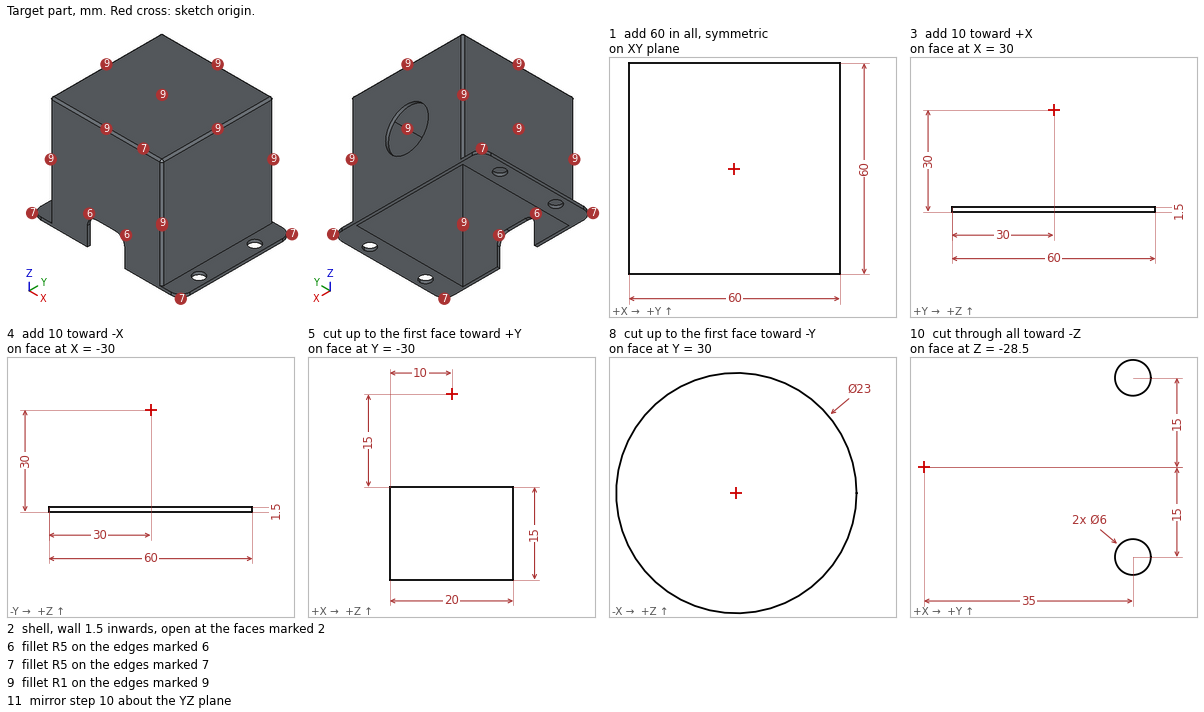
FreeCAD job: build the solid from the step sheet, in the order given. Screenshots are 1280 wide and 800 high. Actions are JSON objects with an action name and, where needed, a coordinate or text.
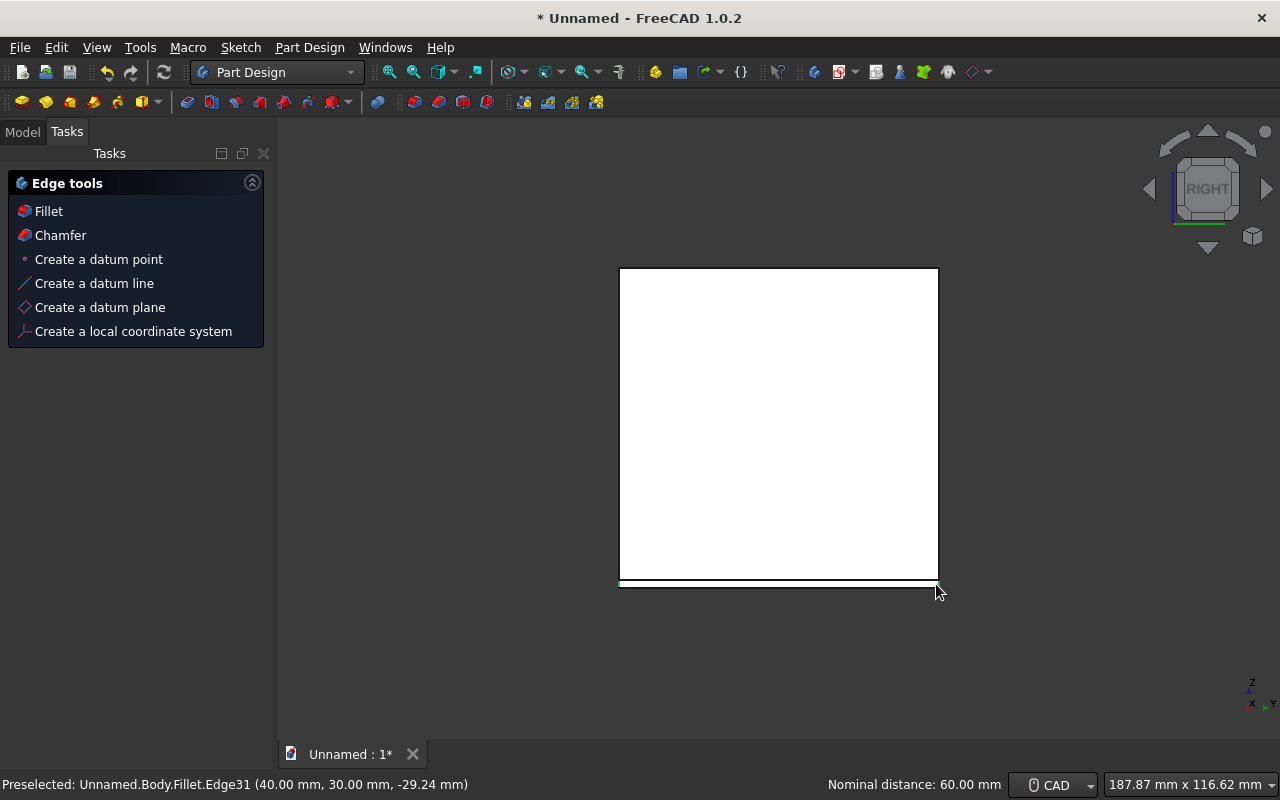
{"action": "key", "text": "5"}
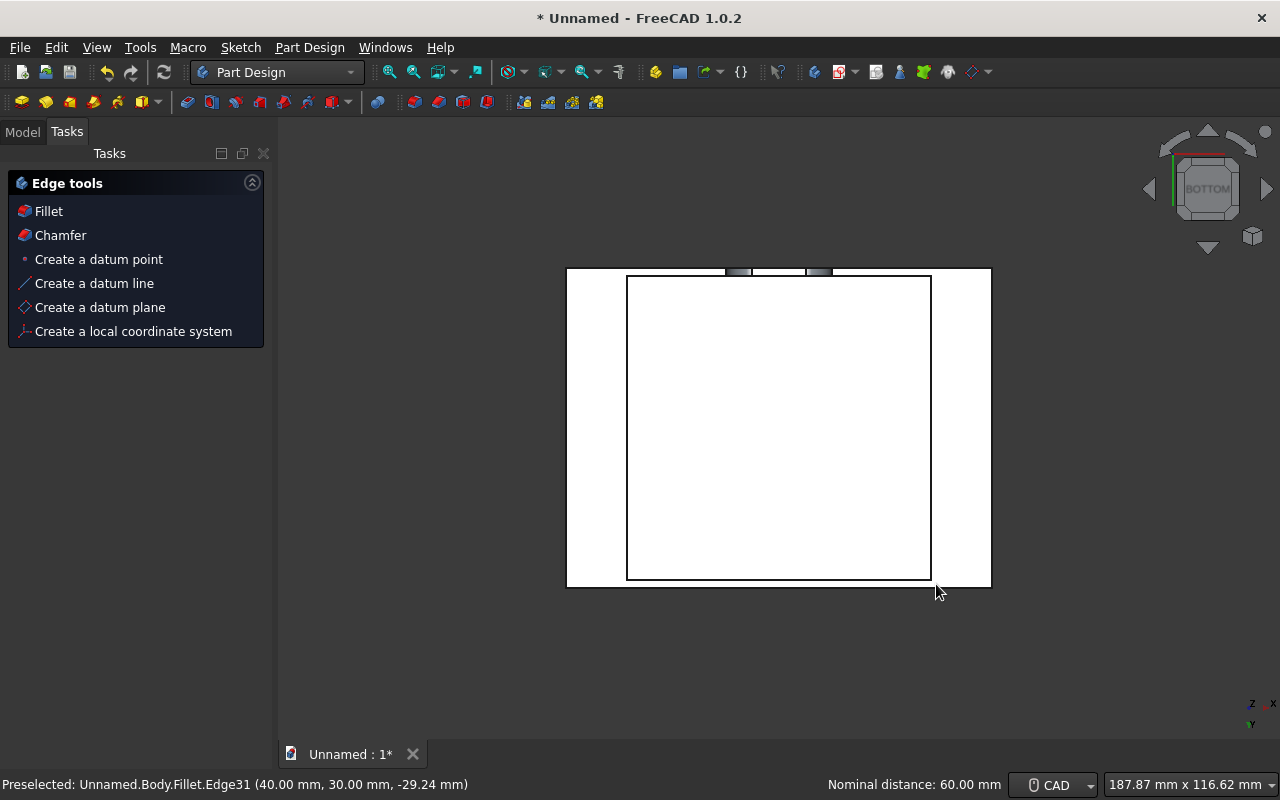
{"action": "scroll", "coordinate": [566, 267], "scroll_direction": "up", "scroll_amount": 9}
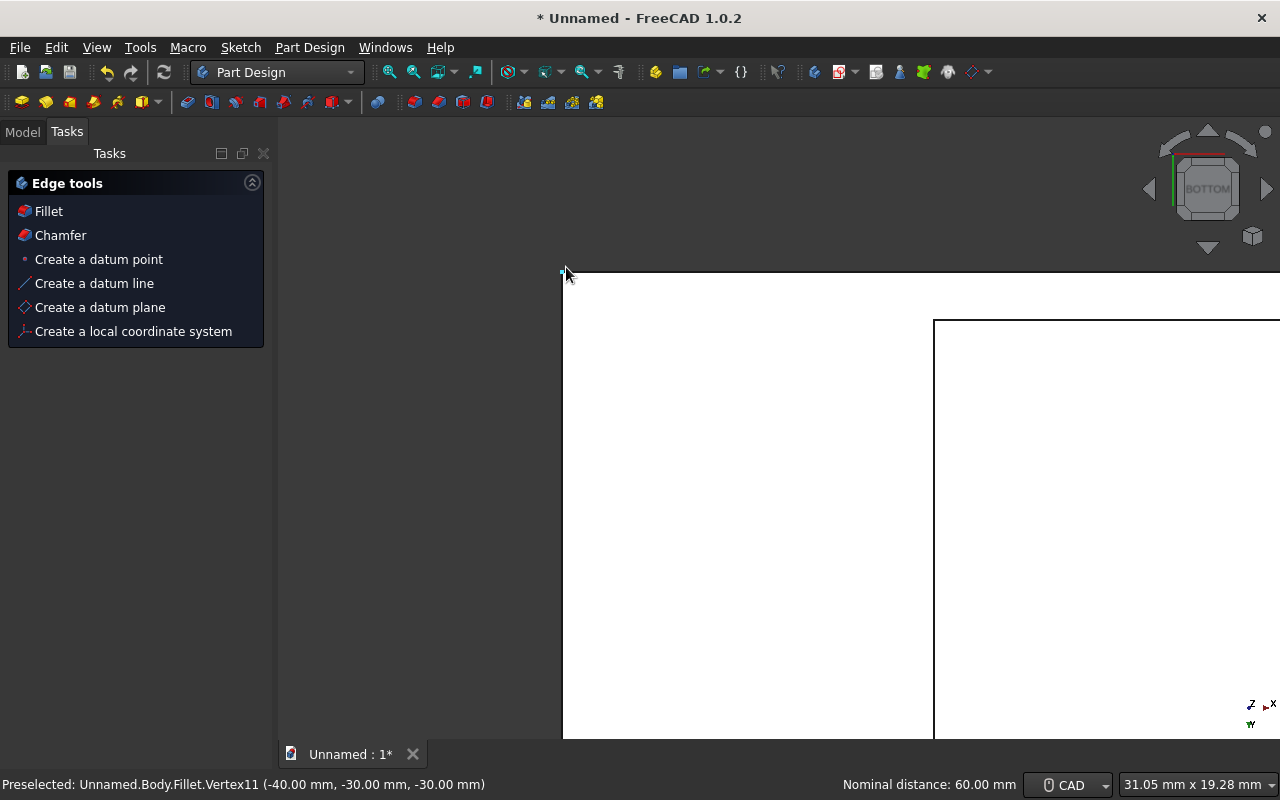
{"action": "key", "text": "v f"}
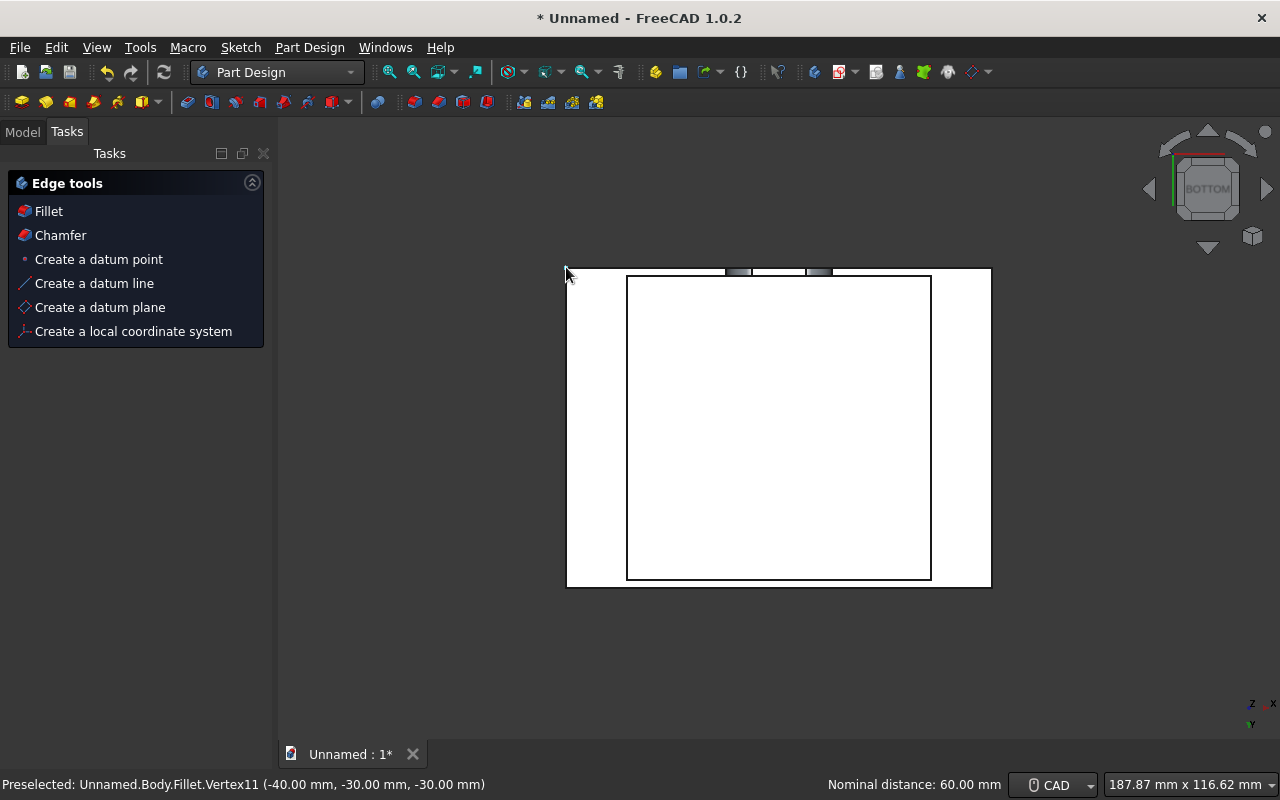
{"action": "key", "text": "4"}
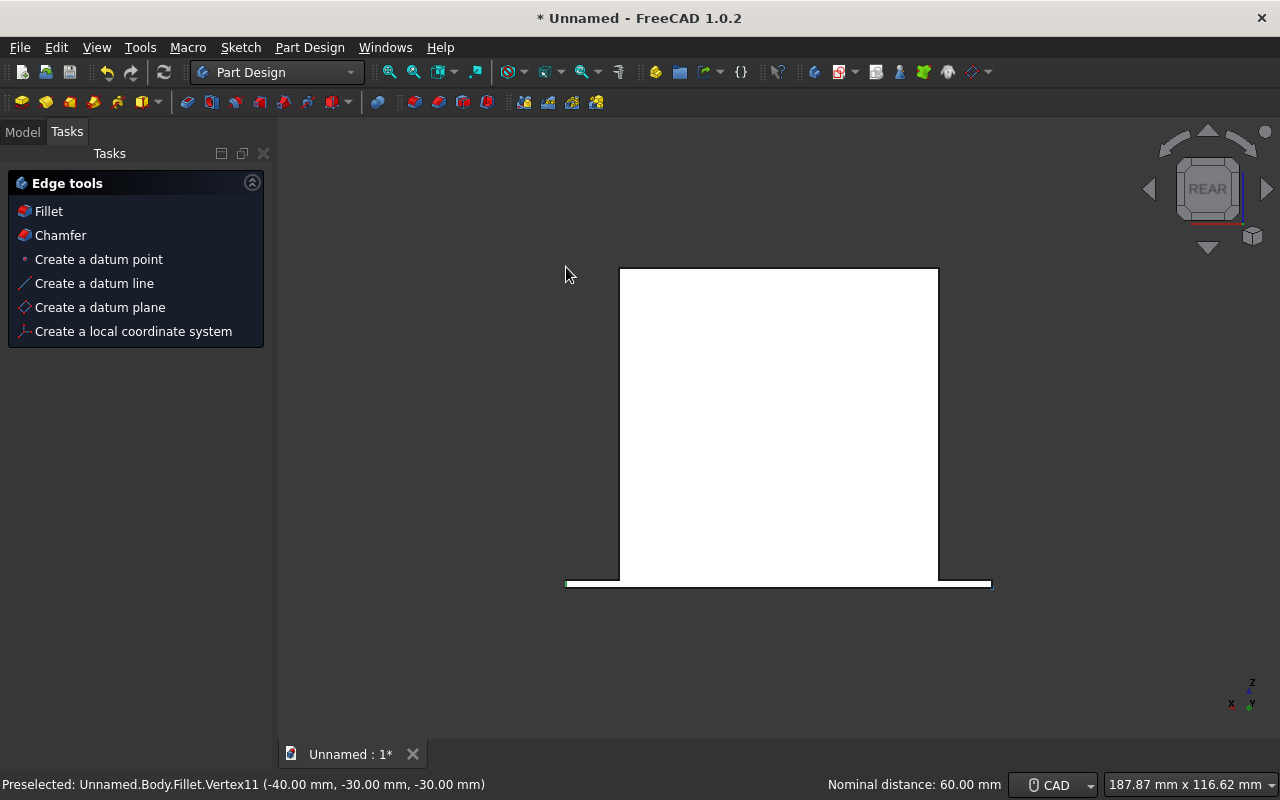
{"action": "scroll", "coordinate": [992, 583], "scroll_direction": "up", "scroll_amount": 9}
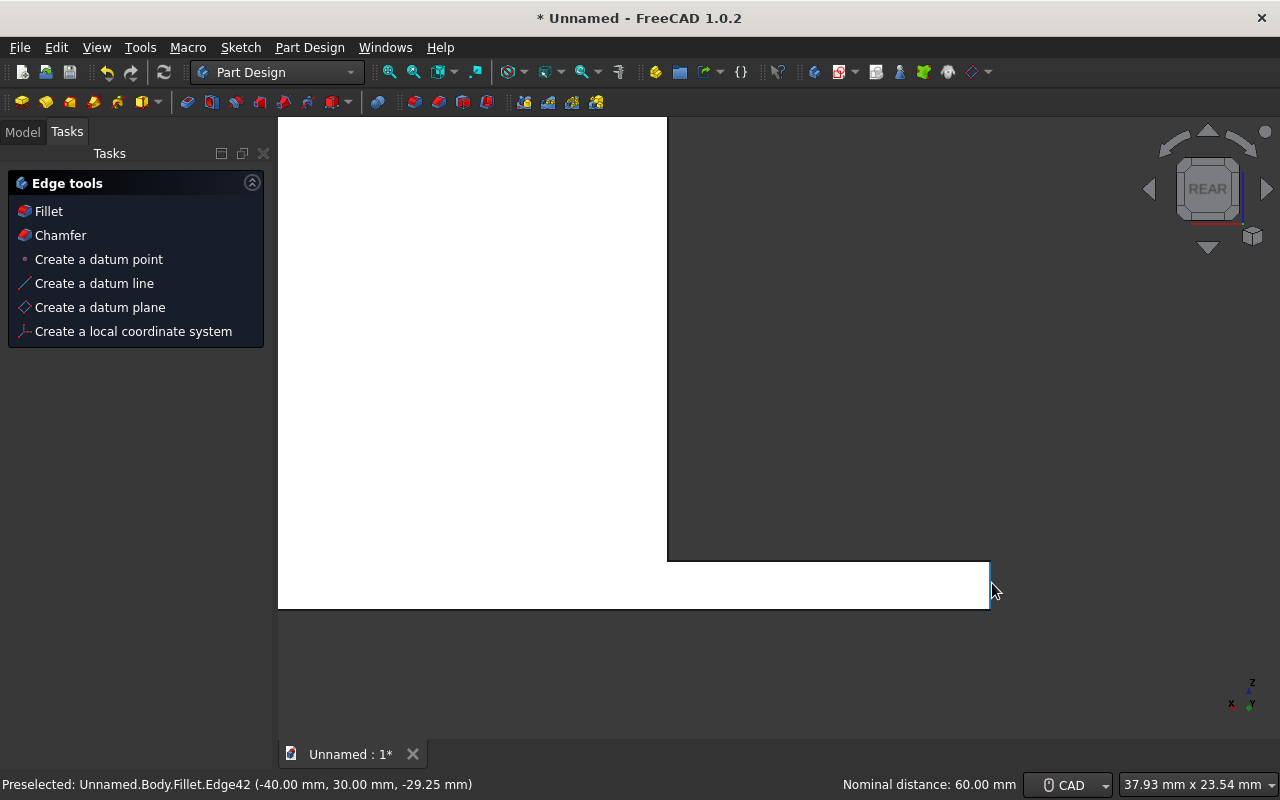
{"action": "left_click", "coordinate": [990, 584], "text": "ctrl"}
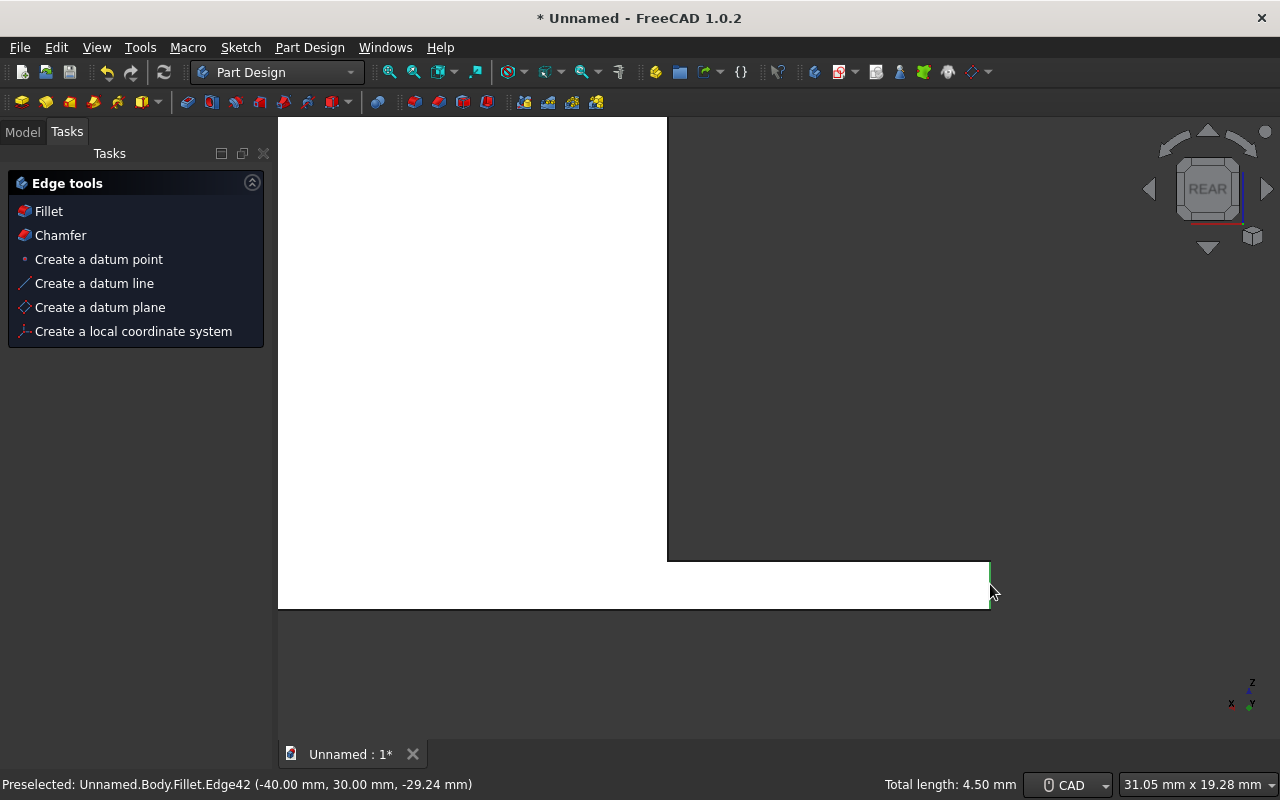
{"action": "left_click", "coordinate": [390, 72]}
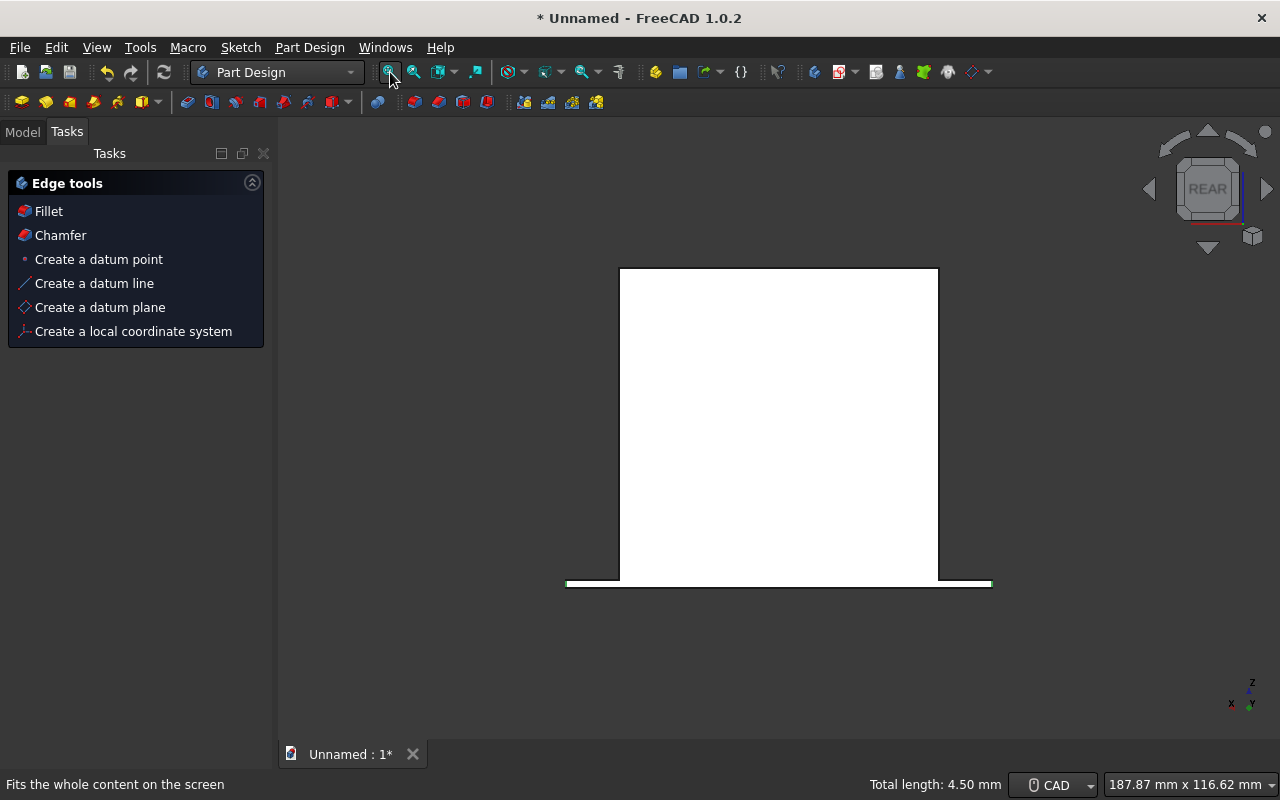
{"action": "key", "text": "6"}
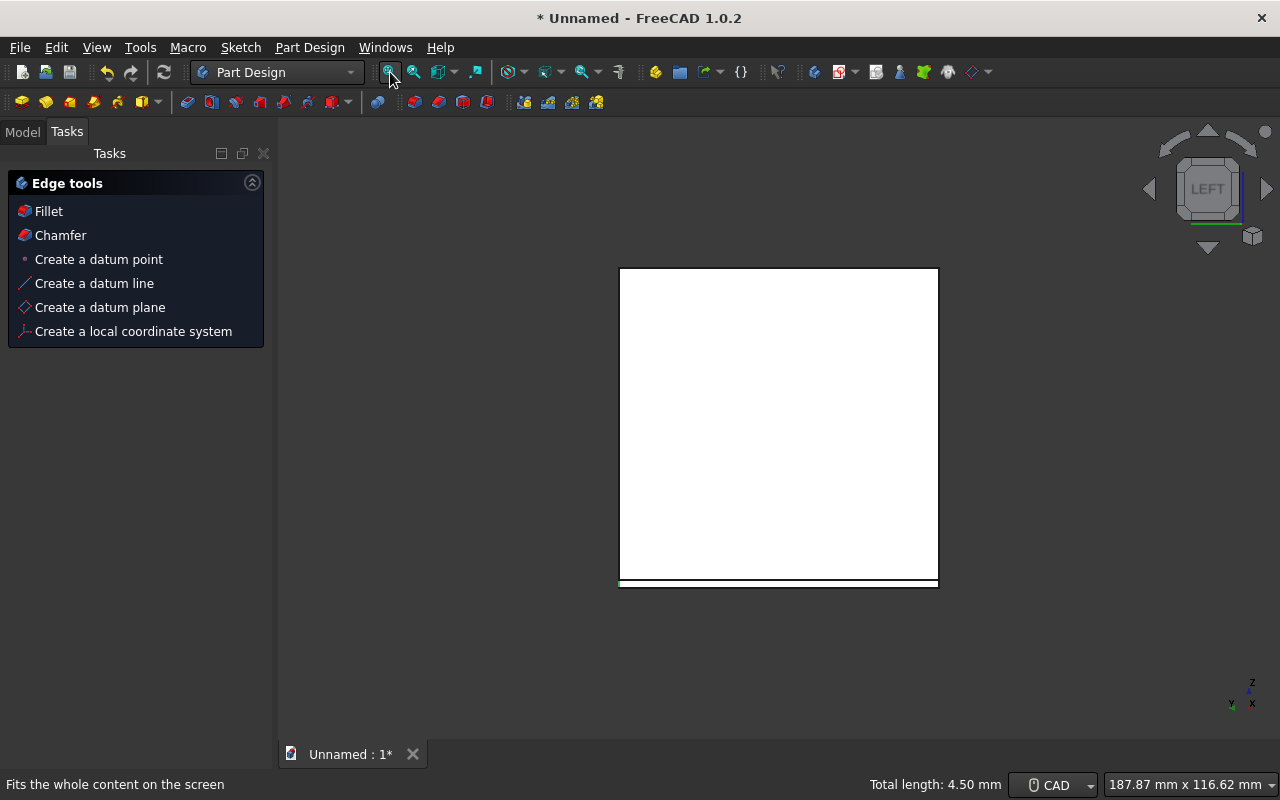
{"action": "scroll", "coordinate": [939, 583], "scroll_direction": "up", "scroll_amount": 9}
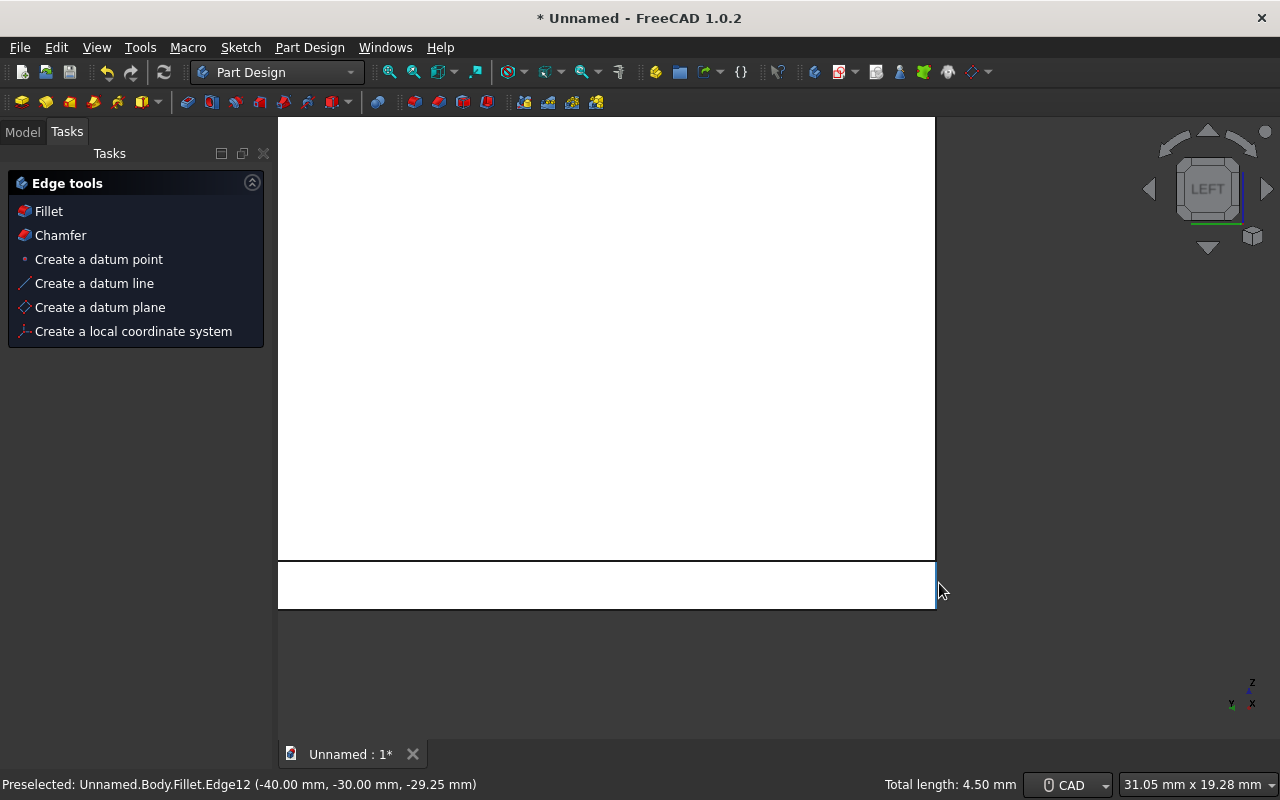
{"action": "left_click", "coordinate": [936, 584], "text": "ctrl"}